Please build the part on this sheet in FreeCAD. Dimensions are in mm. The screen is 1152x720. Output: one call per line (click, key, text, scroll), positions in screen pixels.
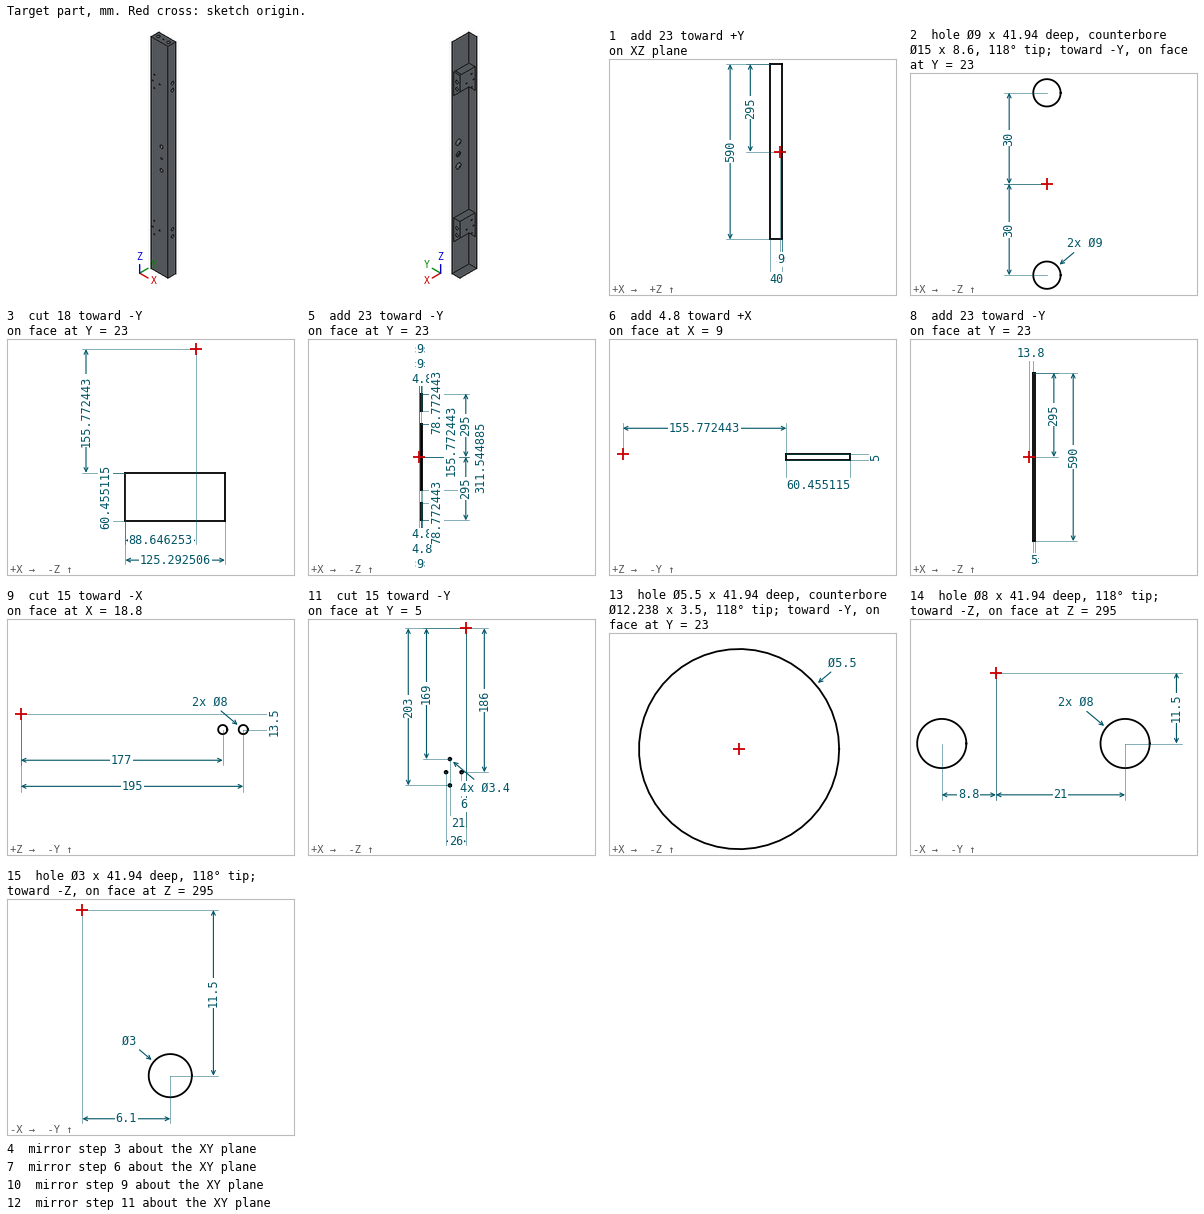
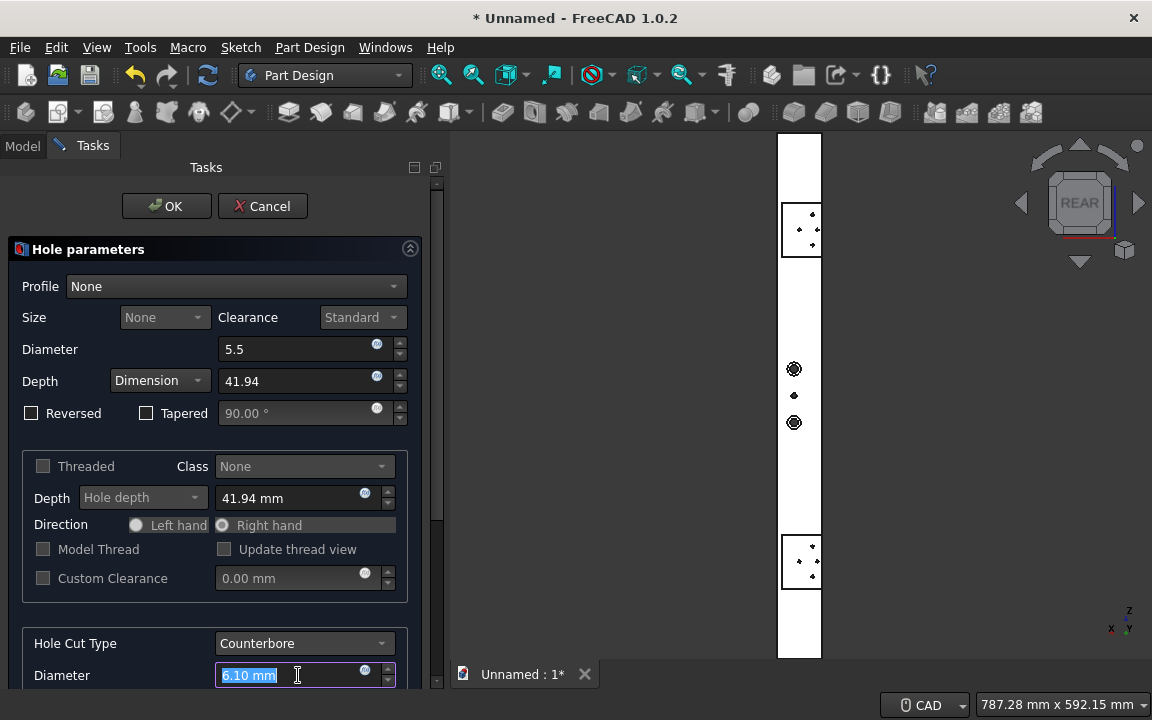
text(12.238)
key(Tab)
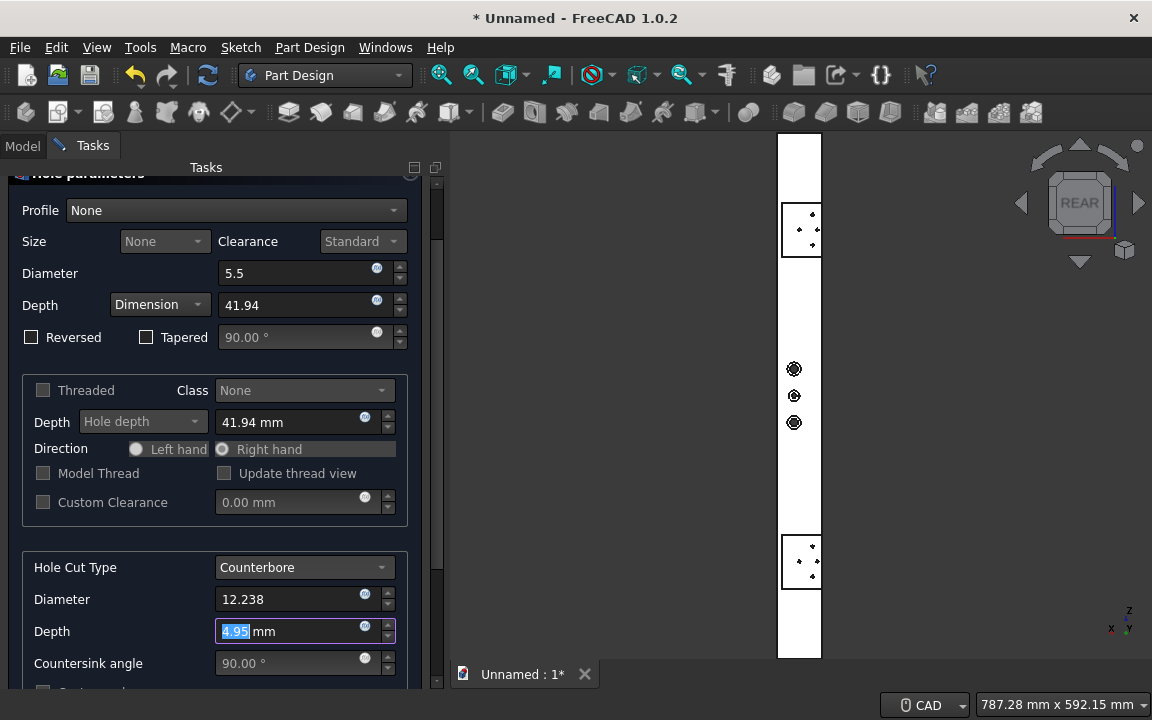
text(3.5)
key(Tab)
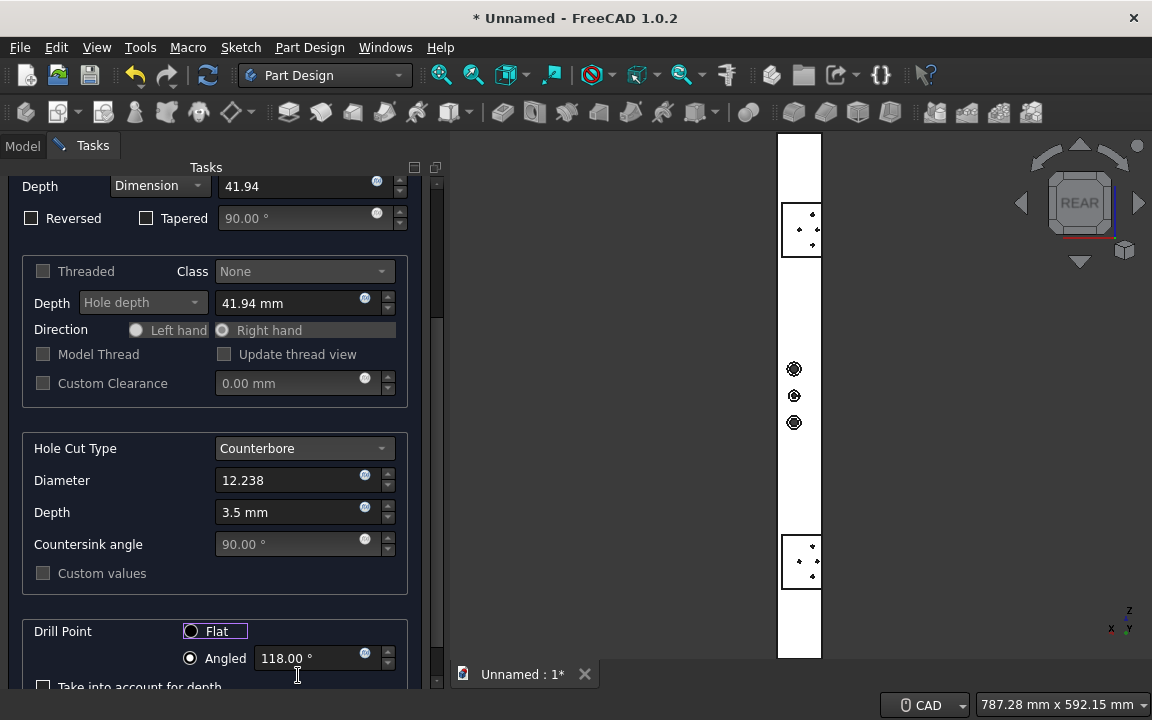
scroll(437, 432, up, 4)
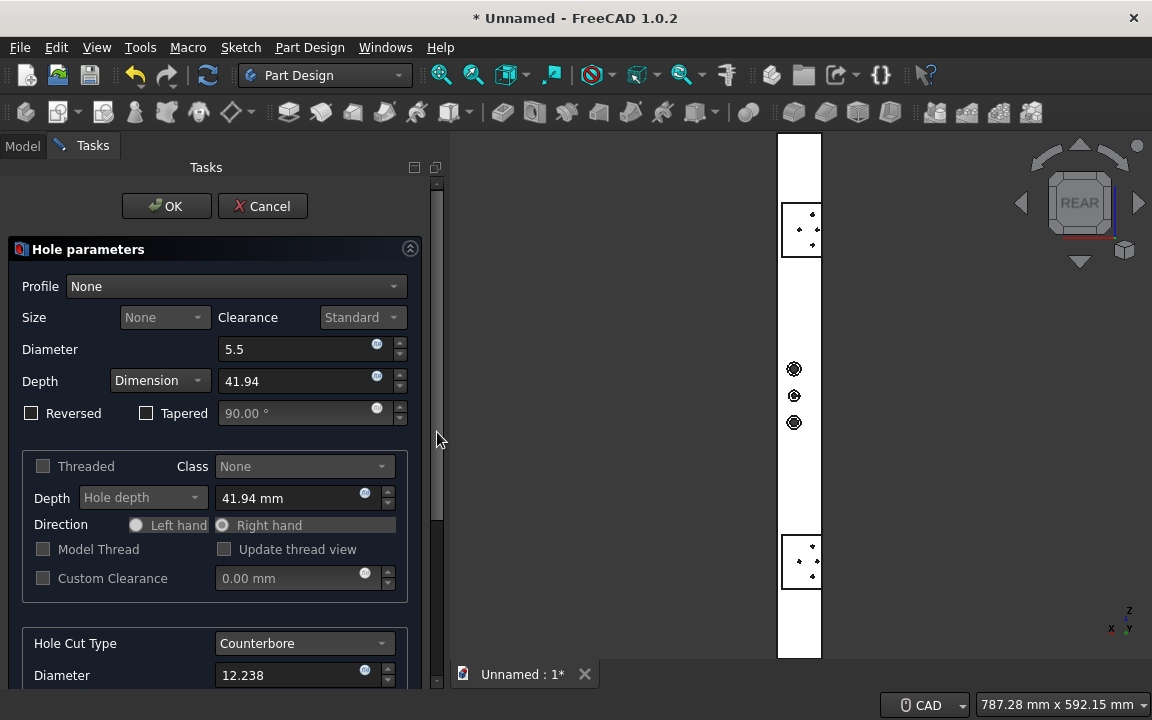
click(167, 206)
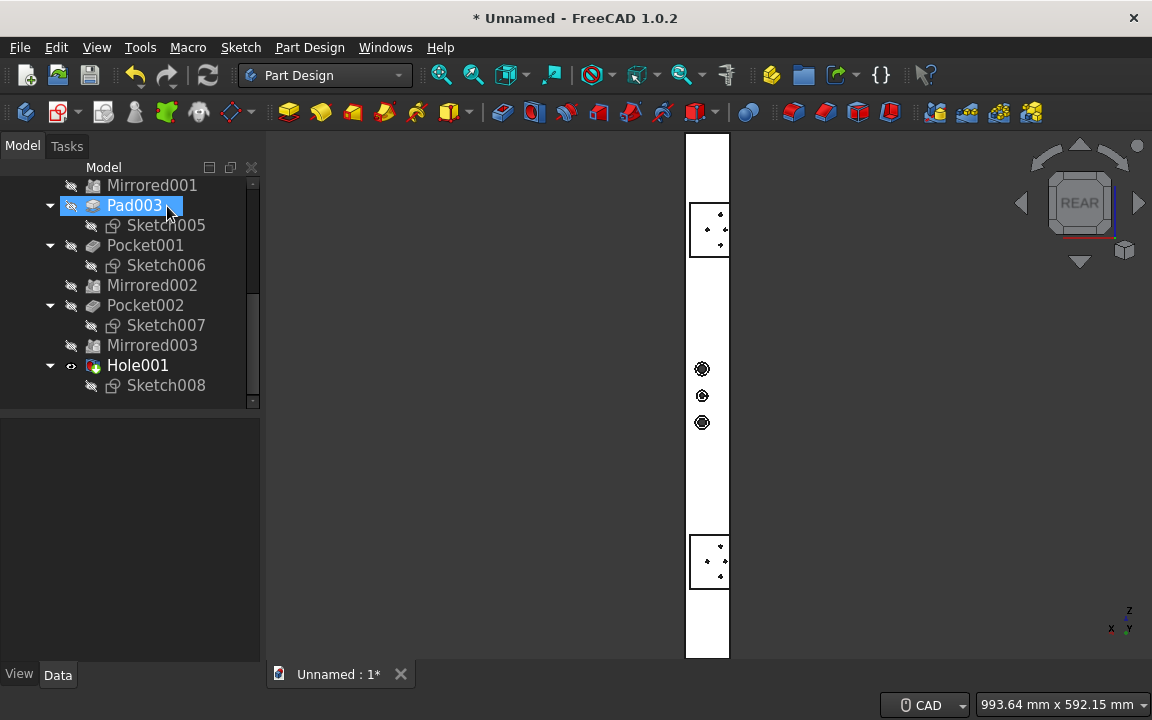
key(0)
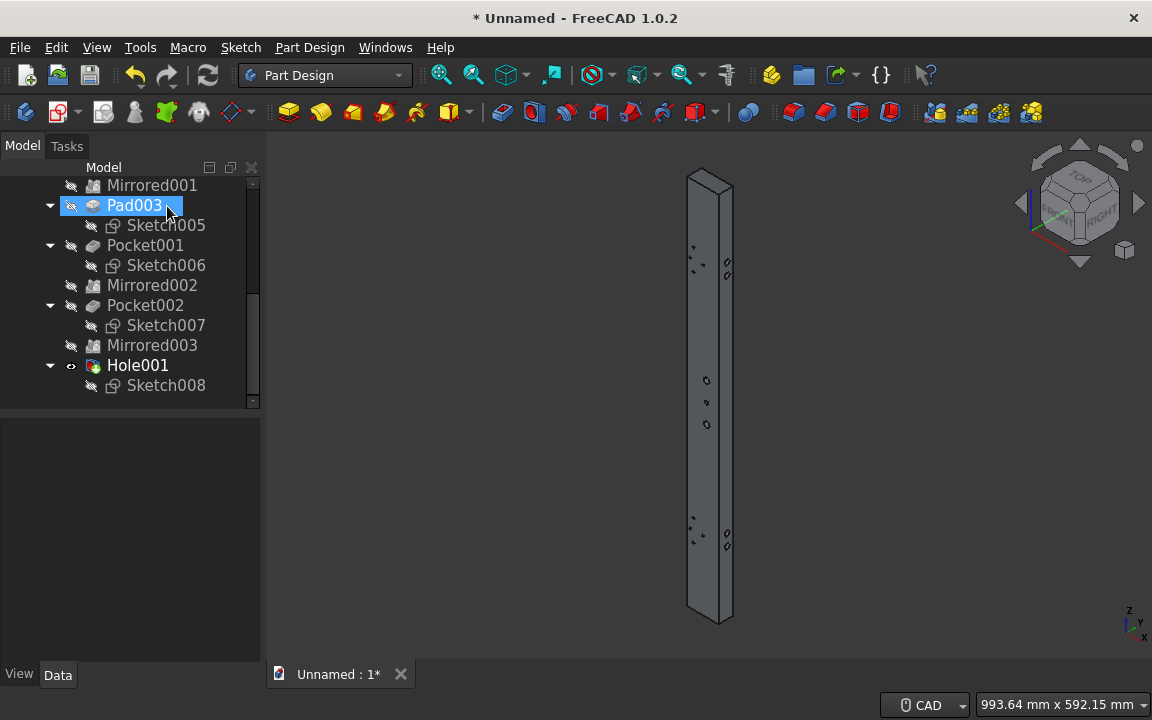
click(717, 182)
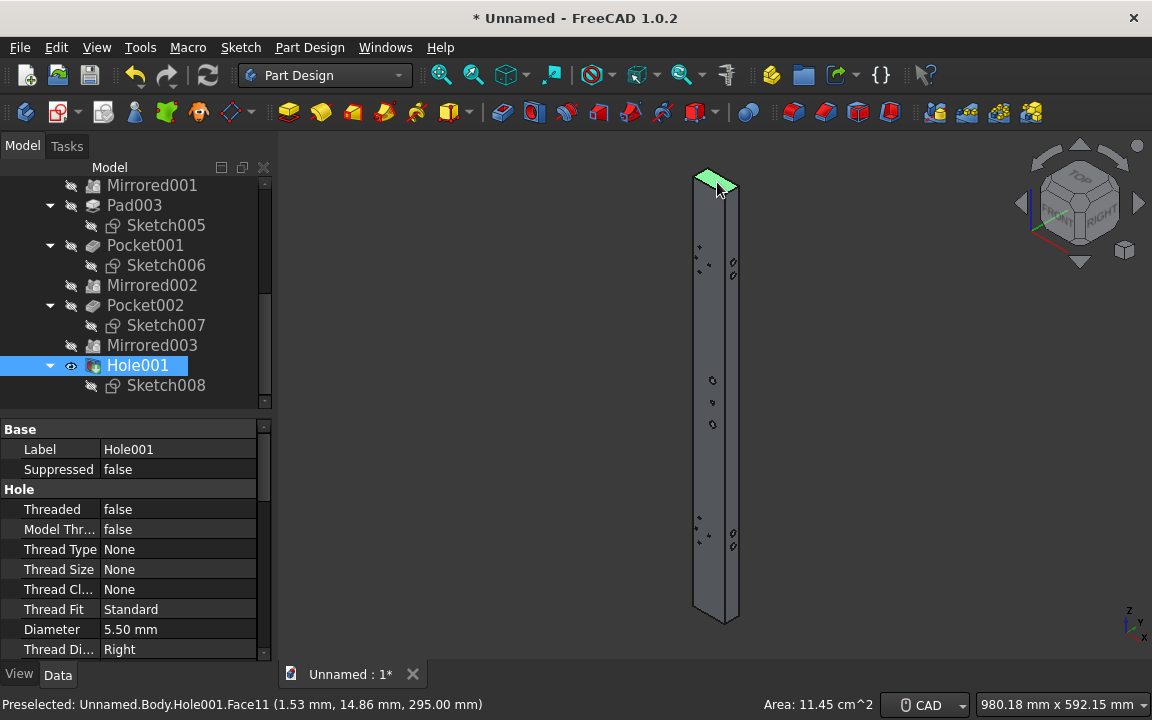
click(58, 112)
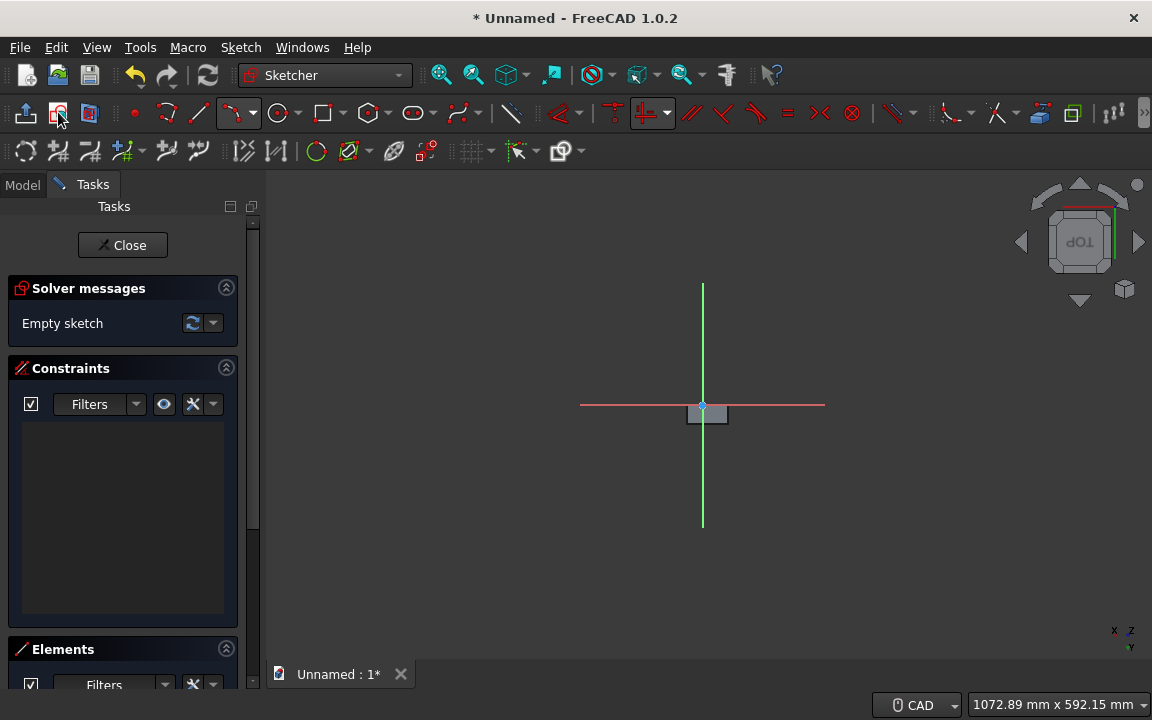
scroll(712, 411, up, 14)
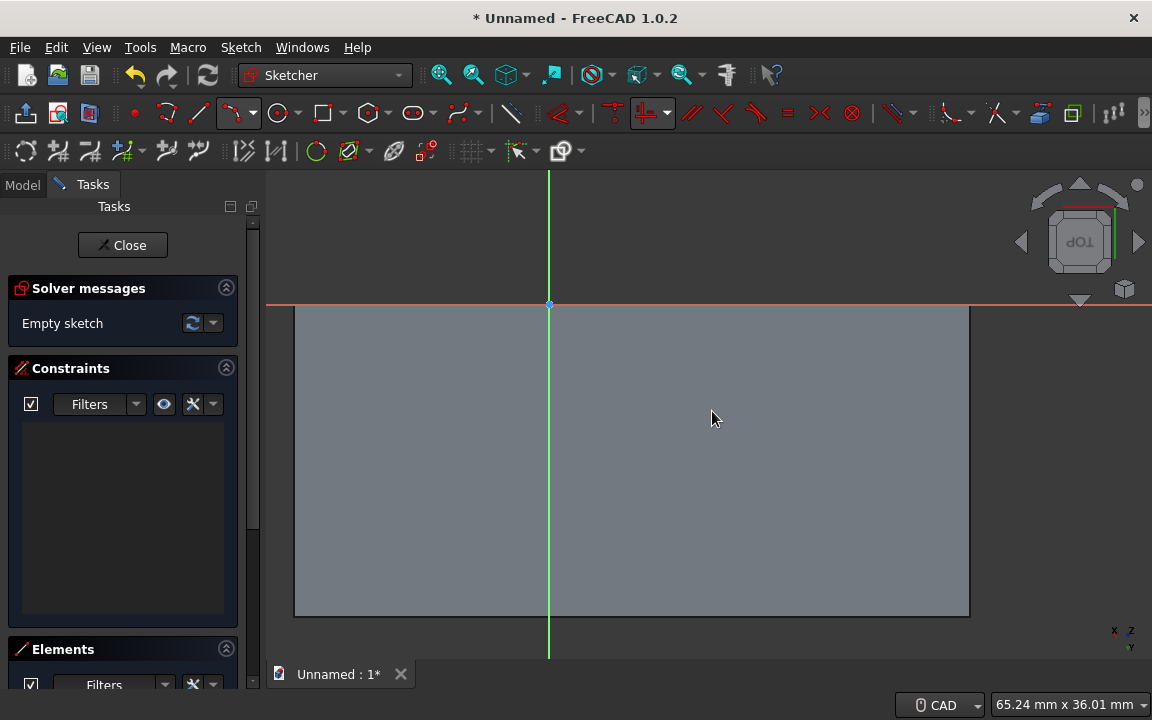
click(278, 114)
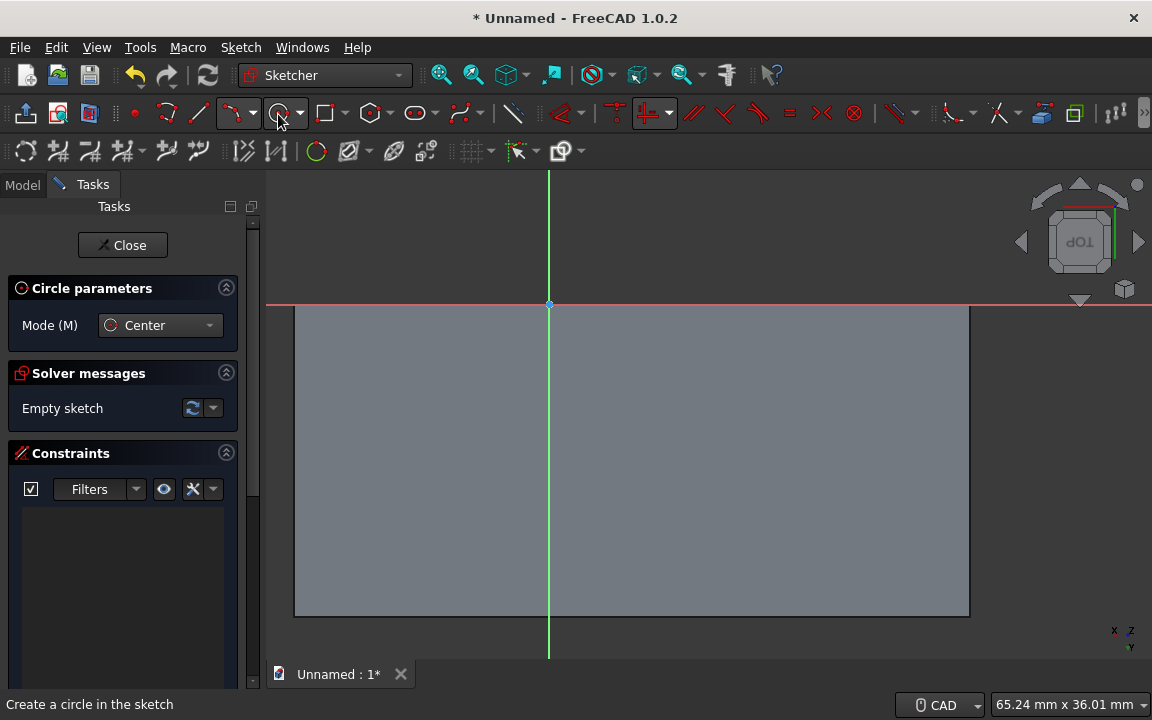
click(834, 461)
click(873, 423)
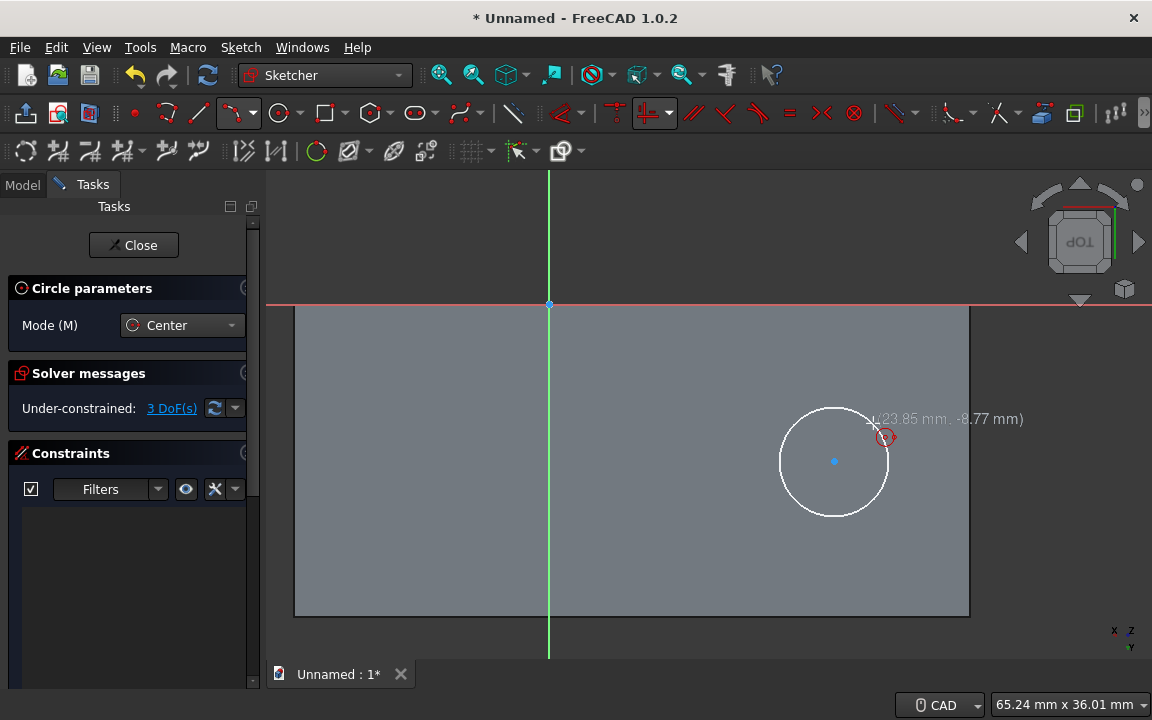
click(430, 461)
click(468, 423)
key(Escape)